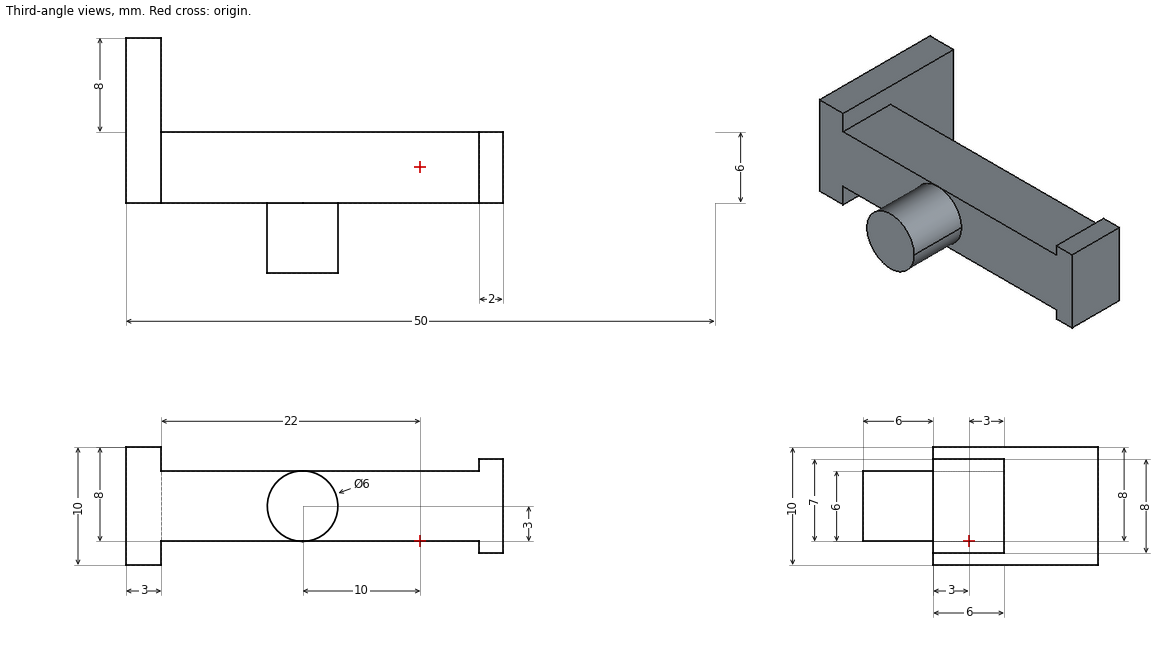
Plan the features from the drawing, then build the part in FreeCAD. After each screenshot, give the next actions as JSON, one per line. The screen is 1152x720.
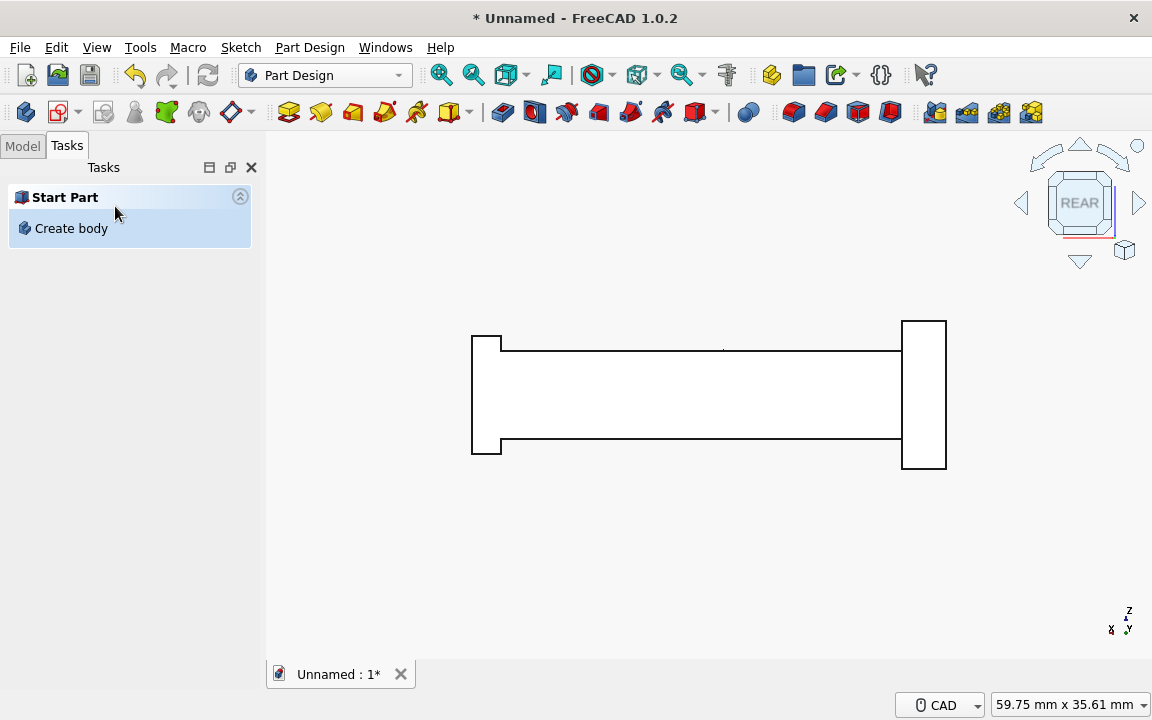
{"action": "key", "text": "0"}